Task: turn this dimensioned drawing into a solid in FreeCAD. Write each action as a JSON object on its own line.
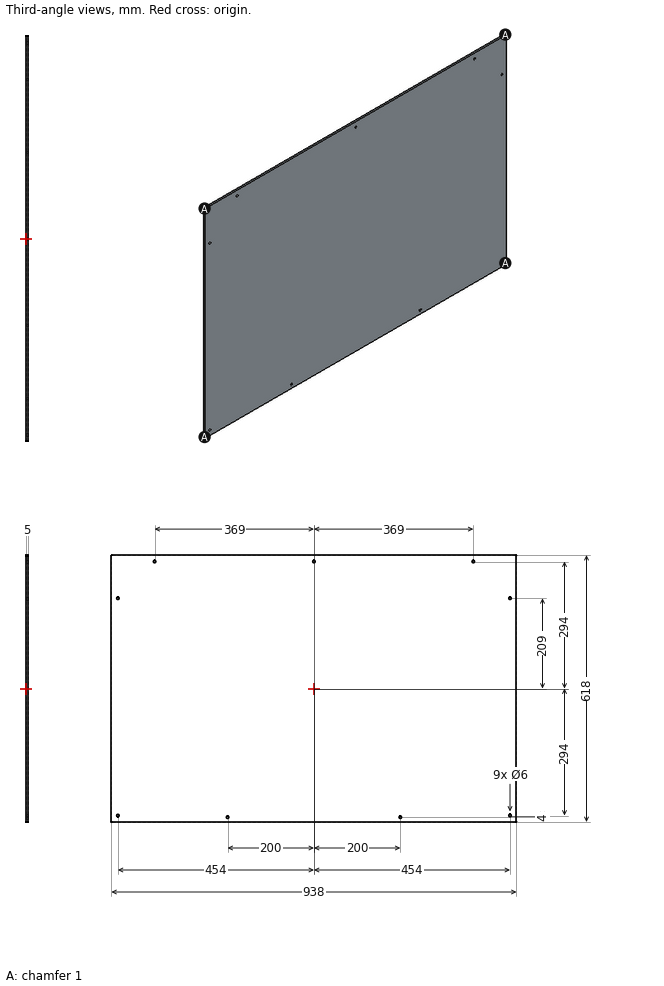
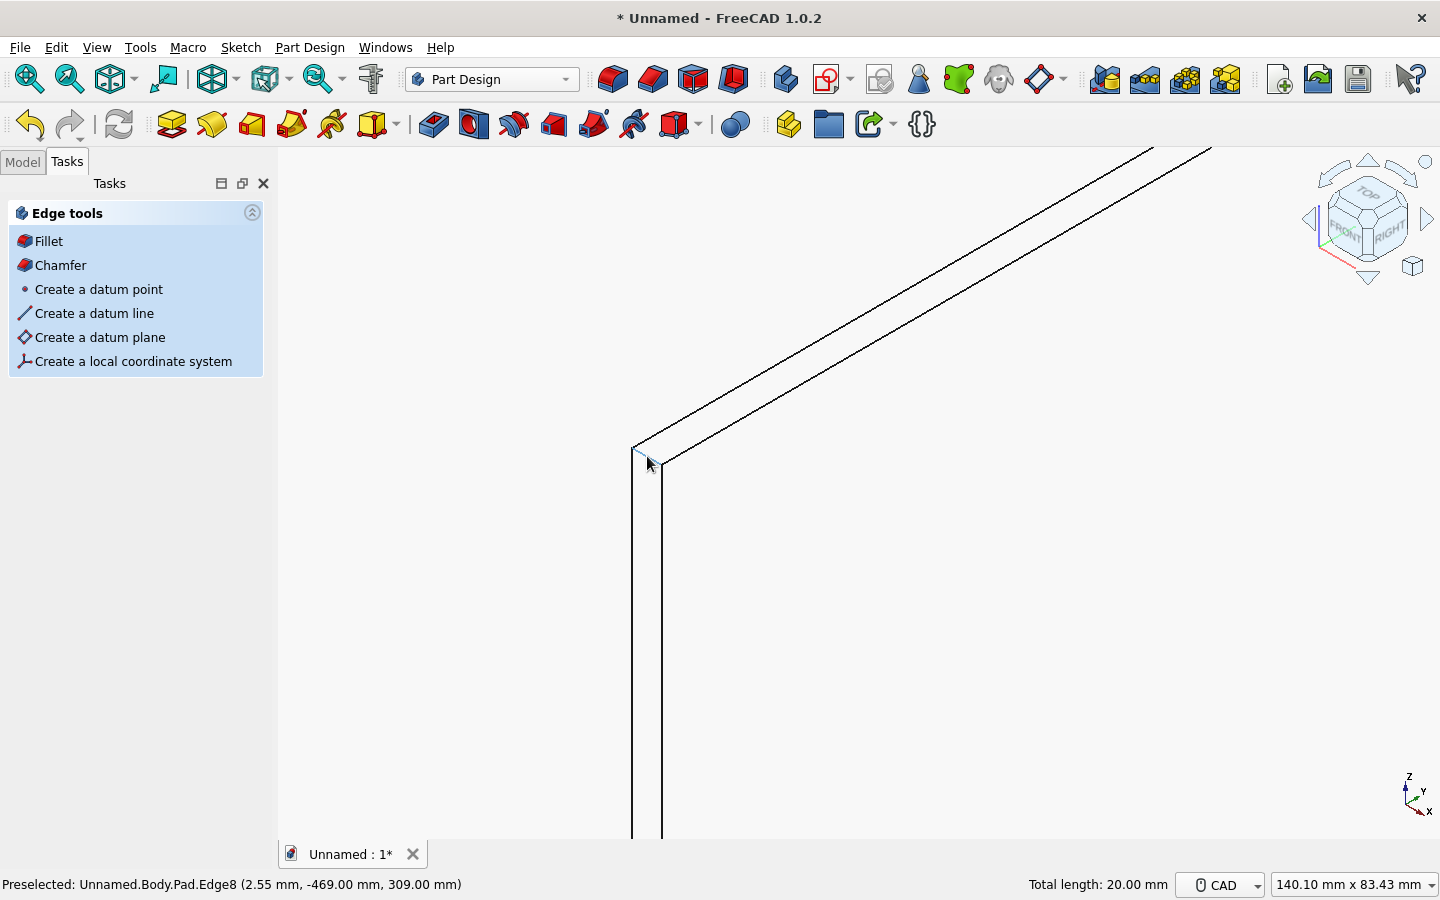
{"action": "key", "text": "v 1"}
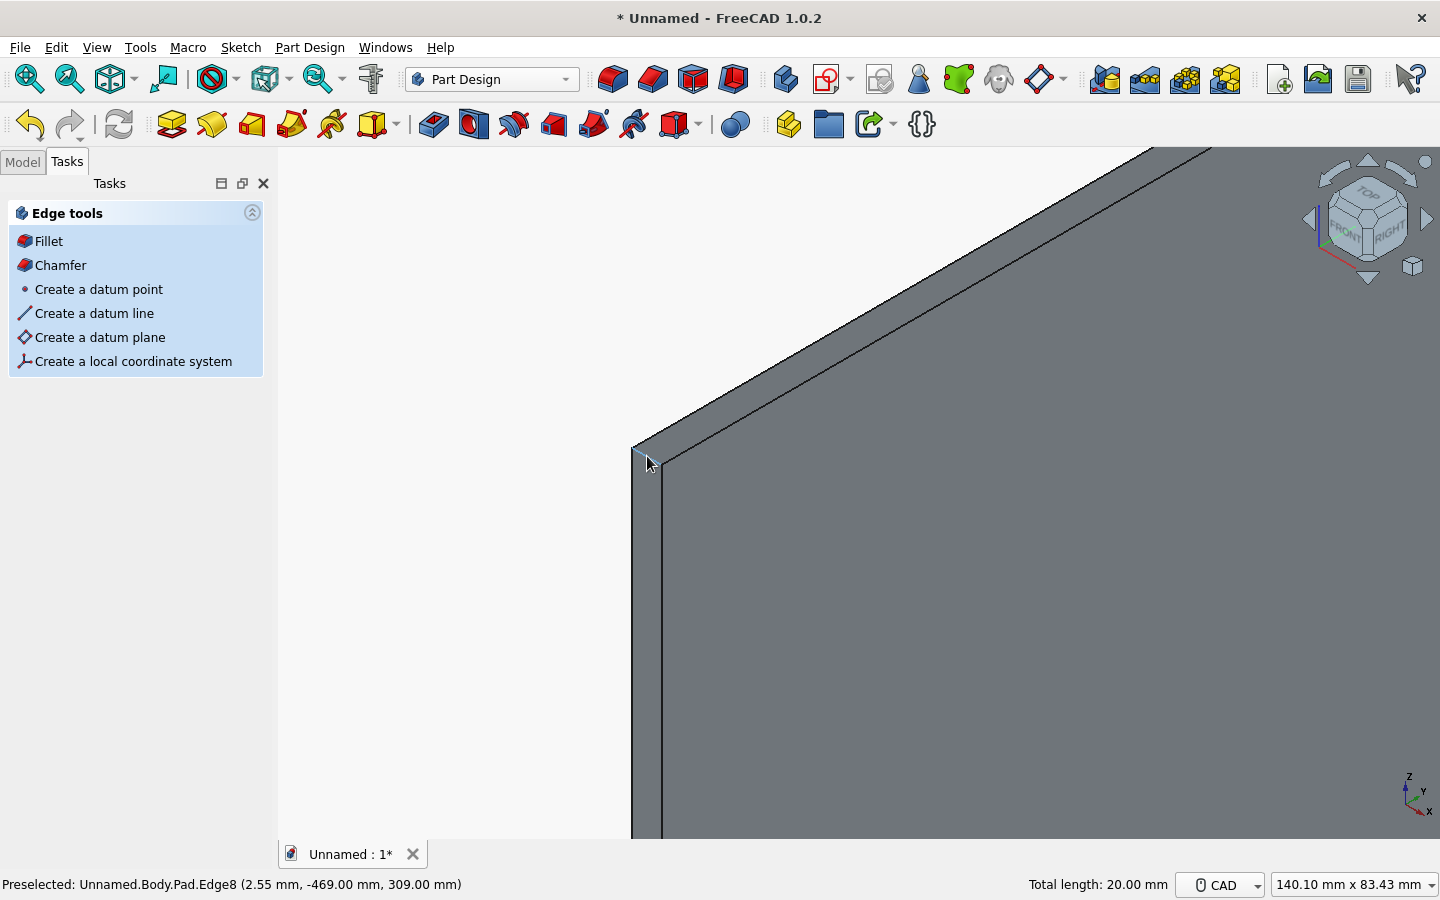
{"action": "left_click", "coordinate": [654, 80]}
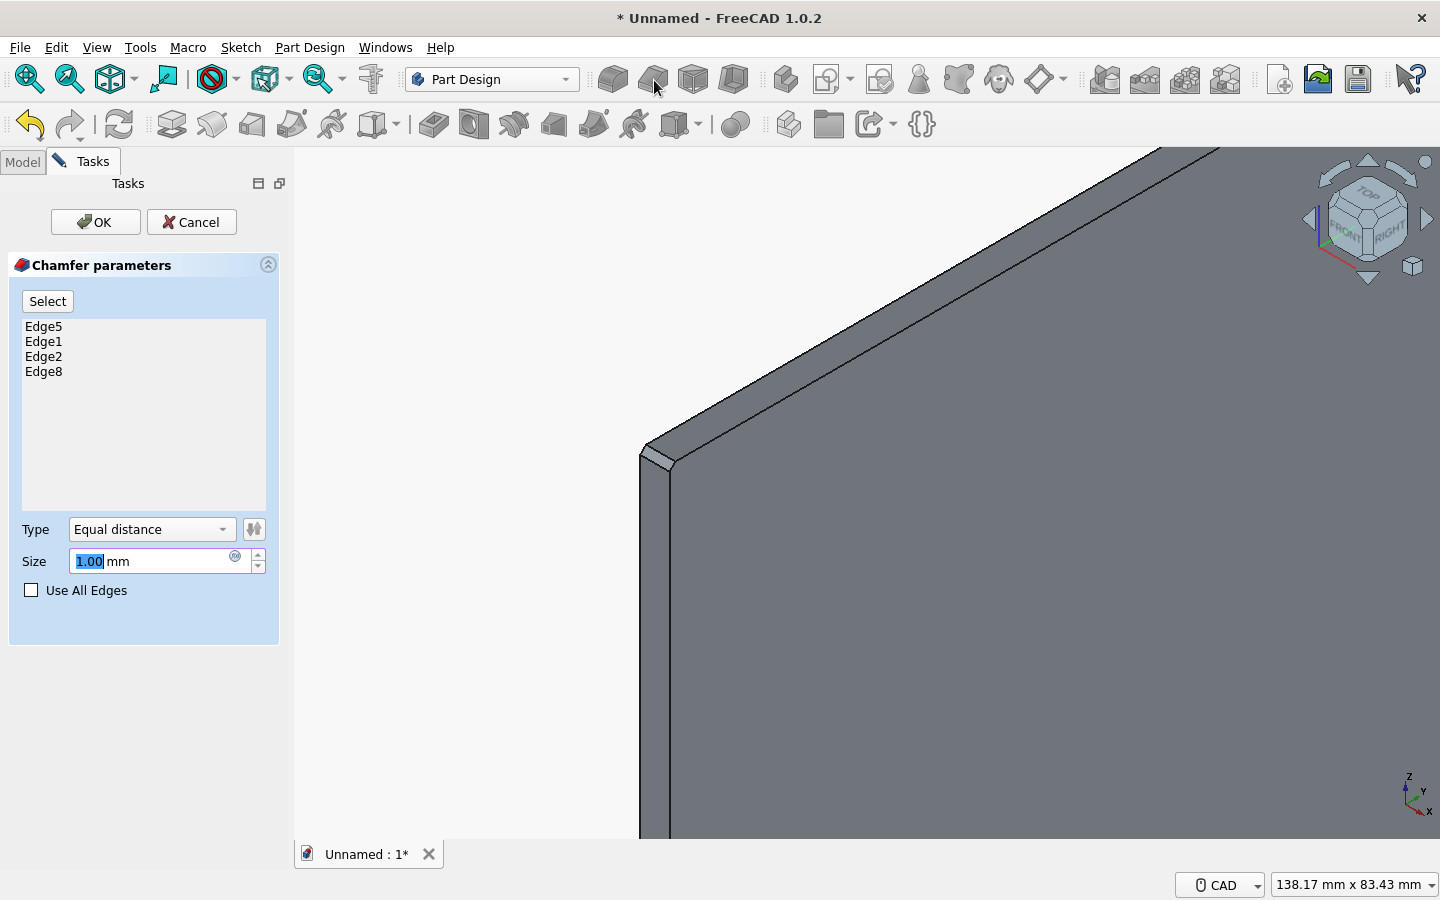
{"action": "type", "text": "1"}
{"action": "key", "text": "Tab"}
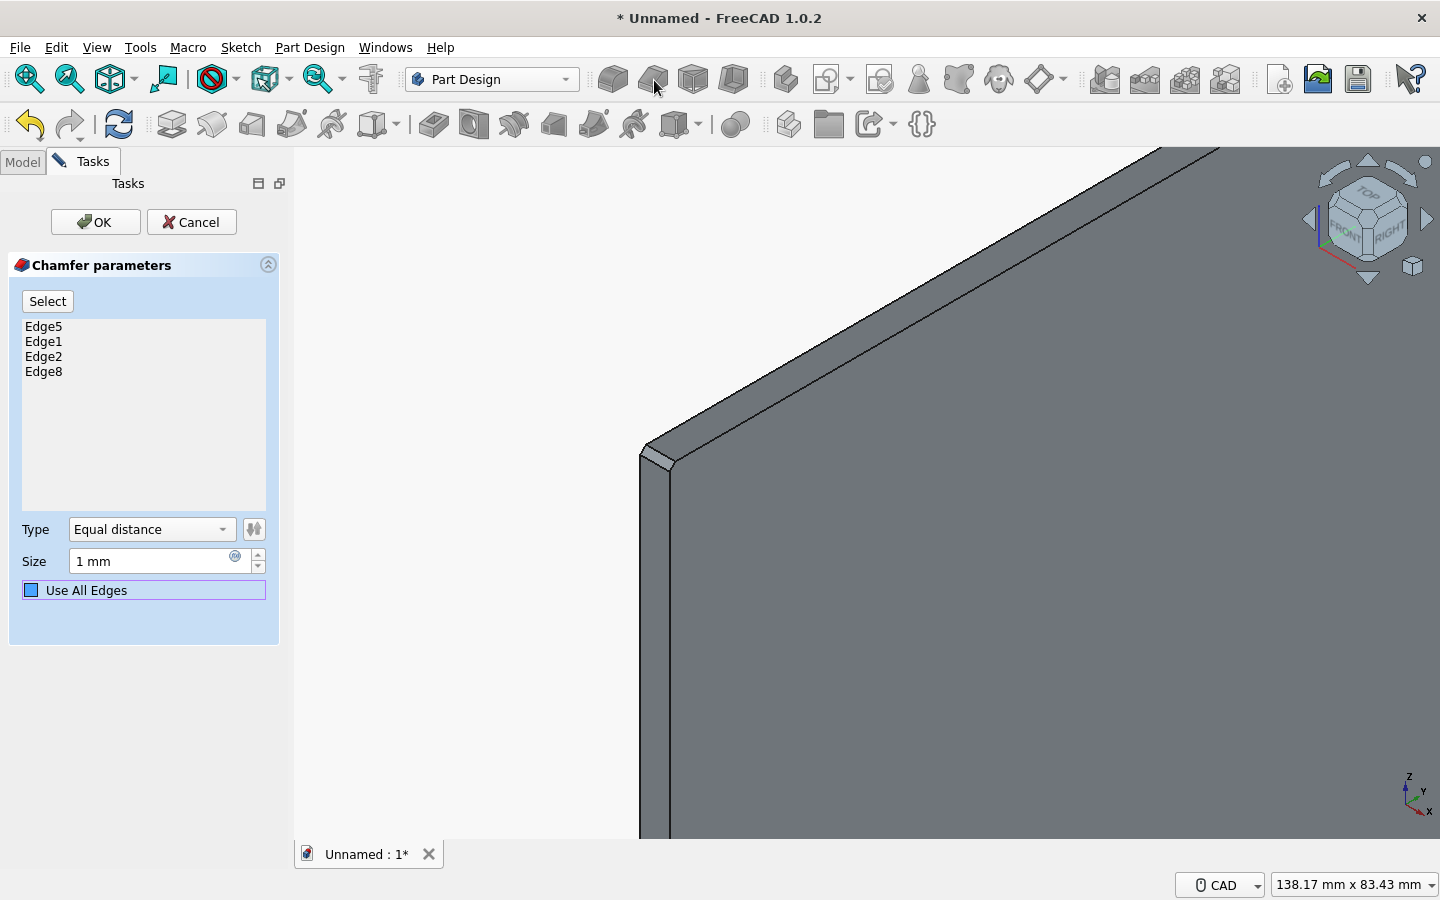
{"action": "left_click", "coordinate": [96, 222]}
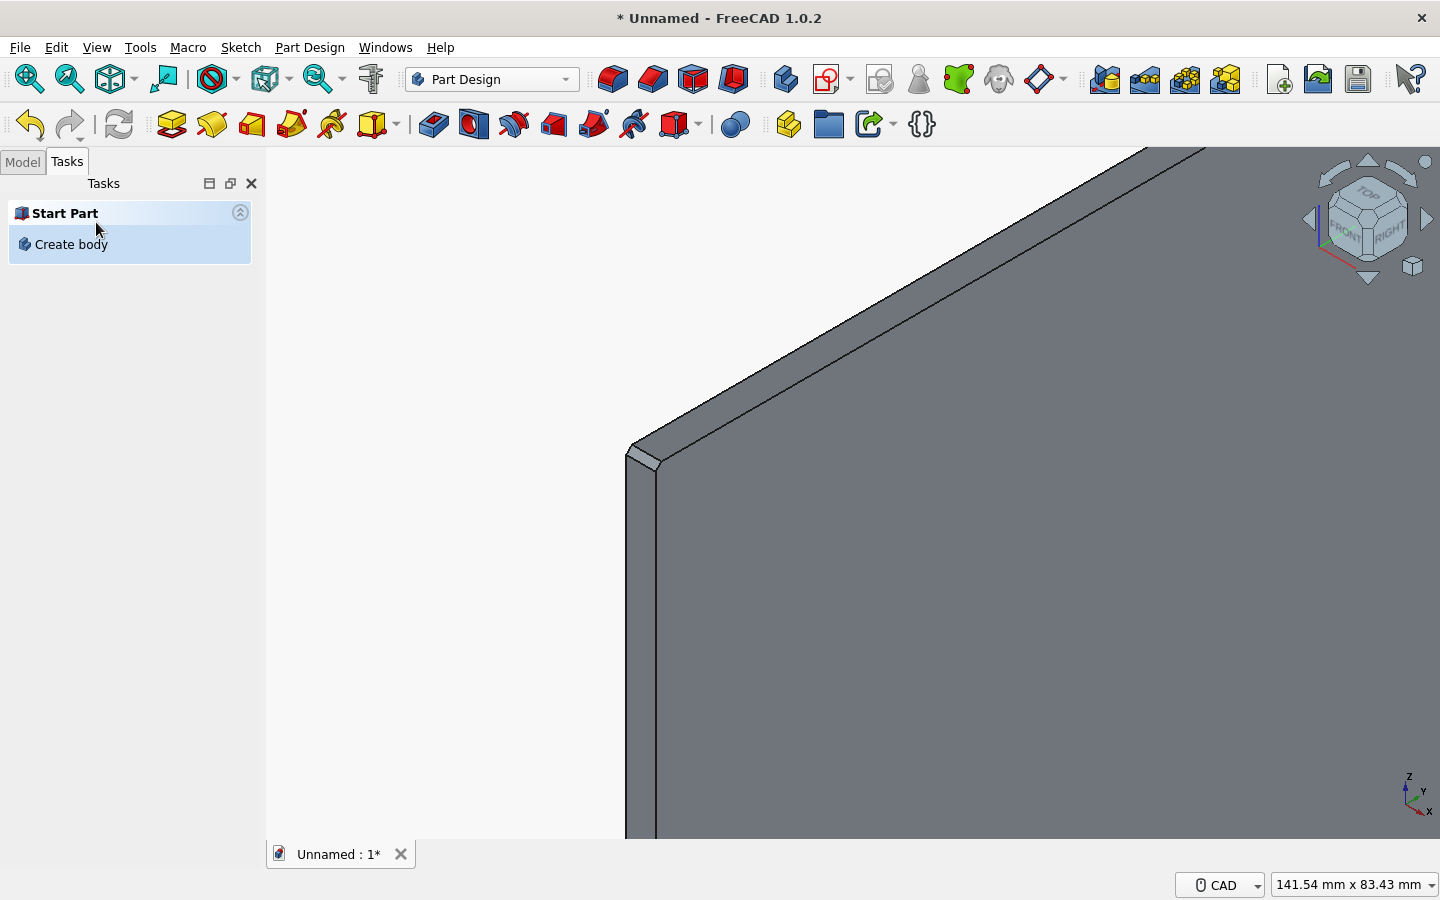
{"action": "key", "text": "v f"}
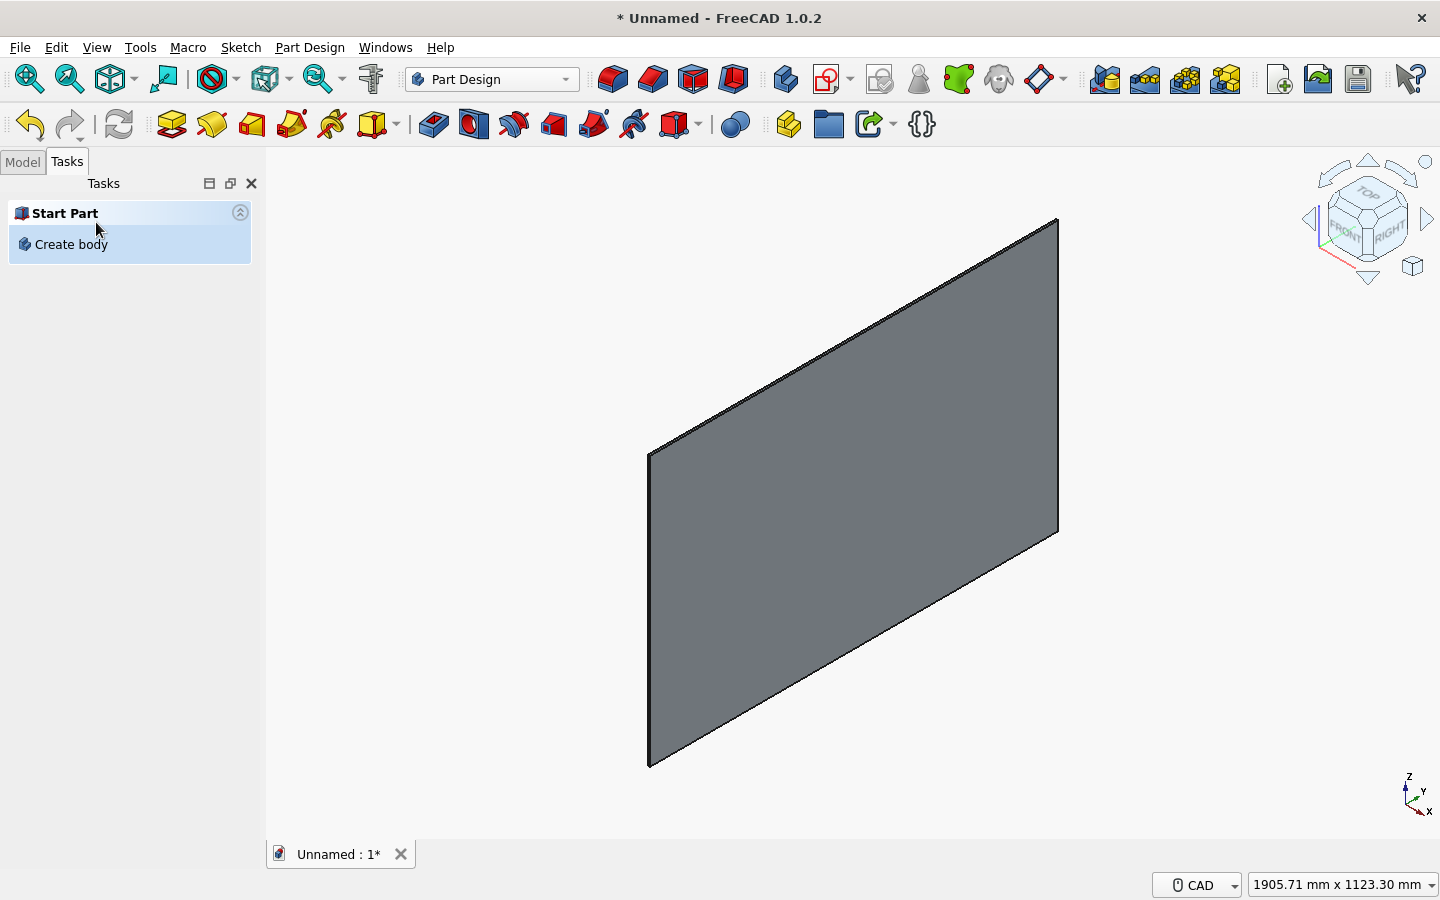
{"action": "key", "text": "6"}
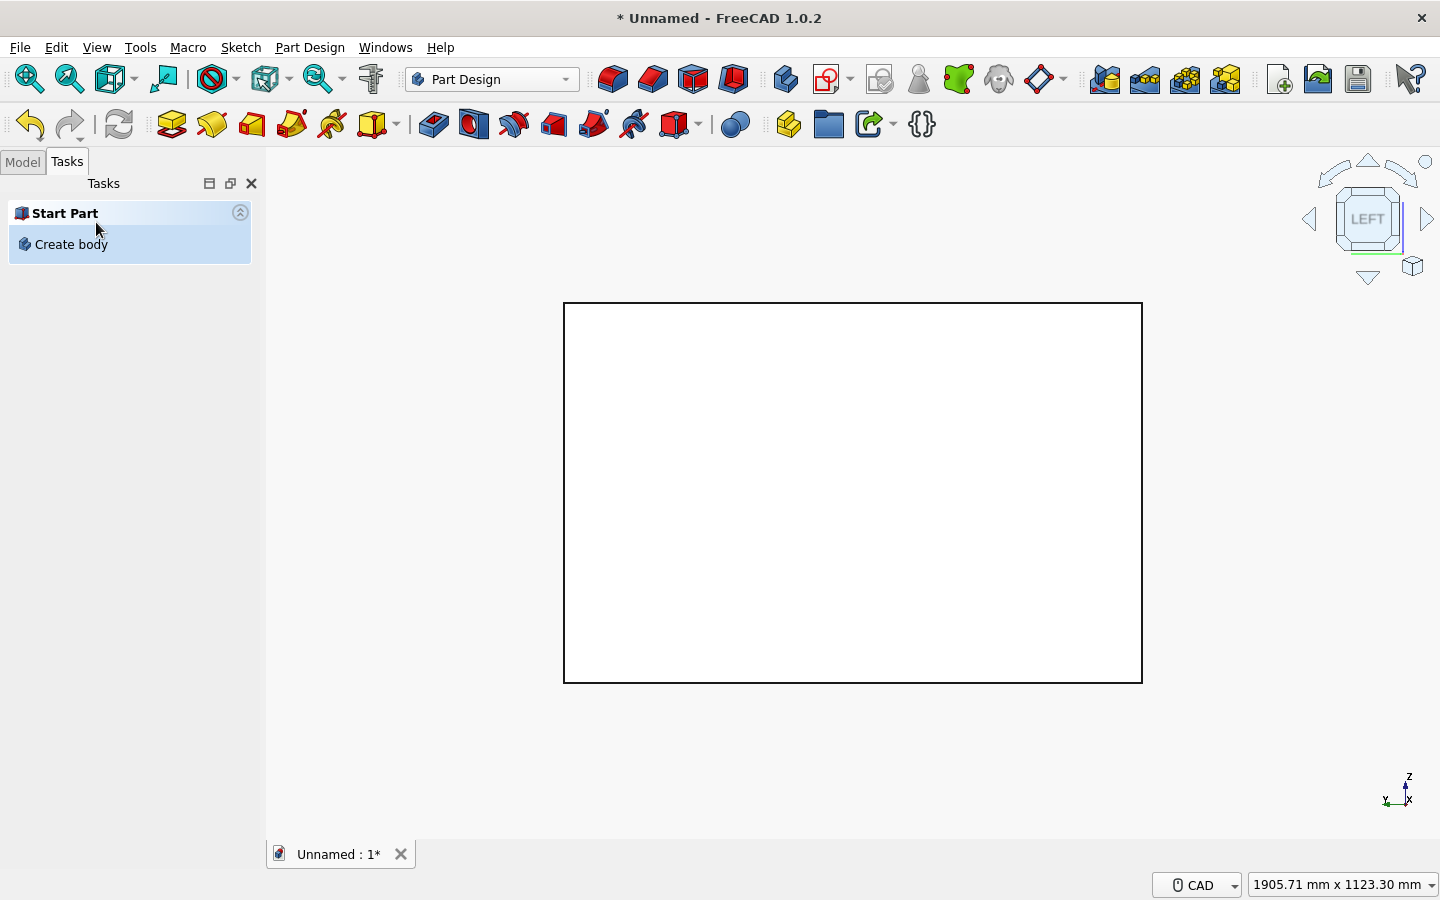
{"action": "left_click", "coordinate": [770, 492]}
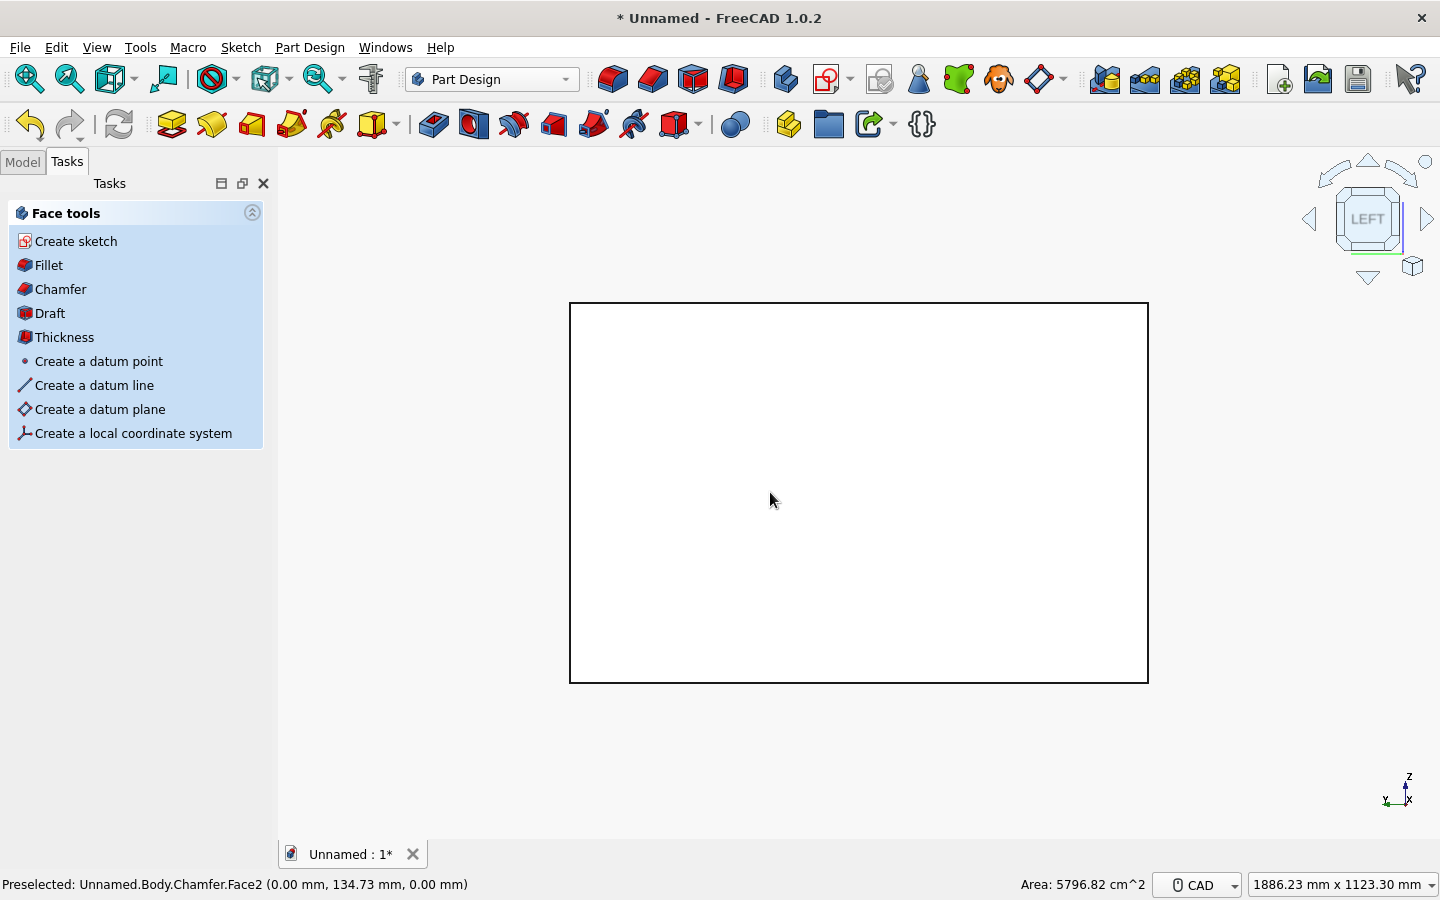
{"action": "left_click", "coordinate": [826, 80]}